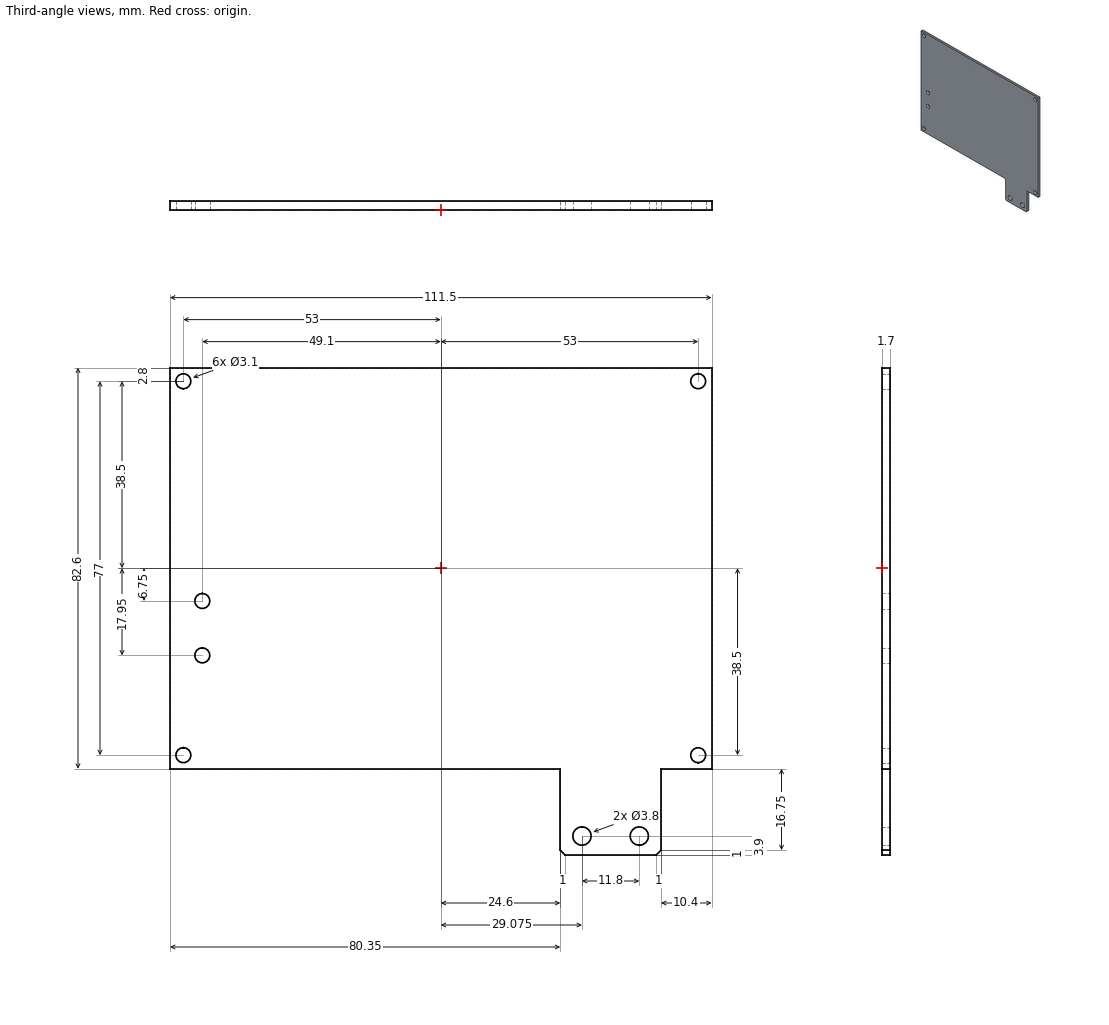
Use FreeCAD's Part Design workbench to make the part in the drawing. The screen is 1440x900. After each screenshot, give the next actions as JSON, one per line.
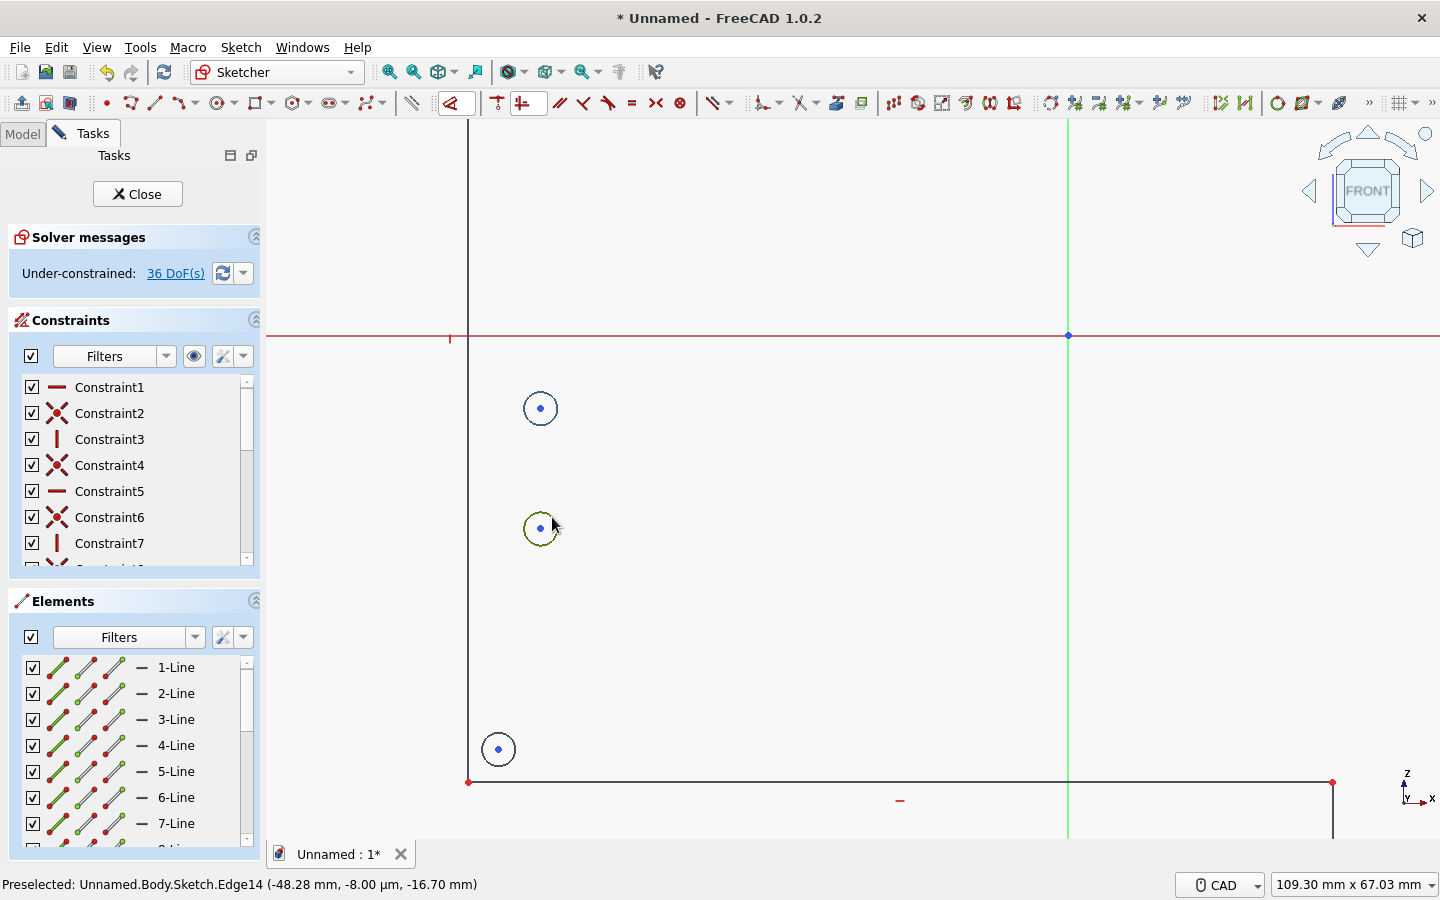
{"action": "left_click", "coordinate": [510, 738]}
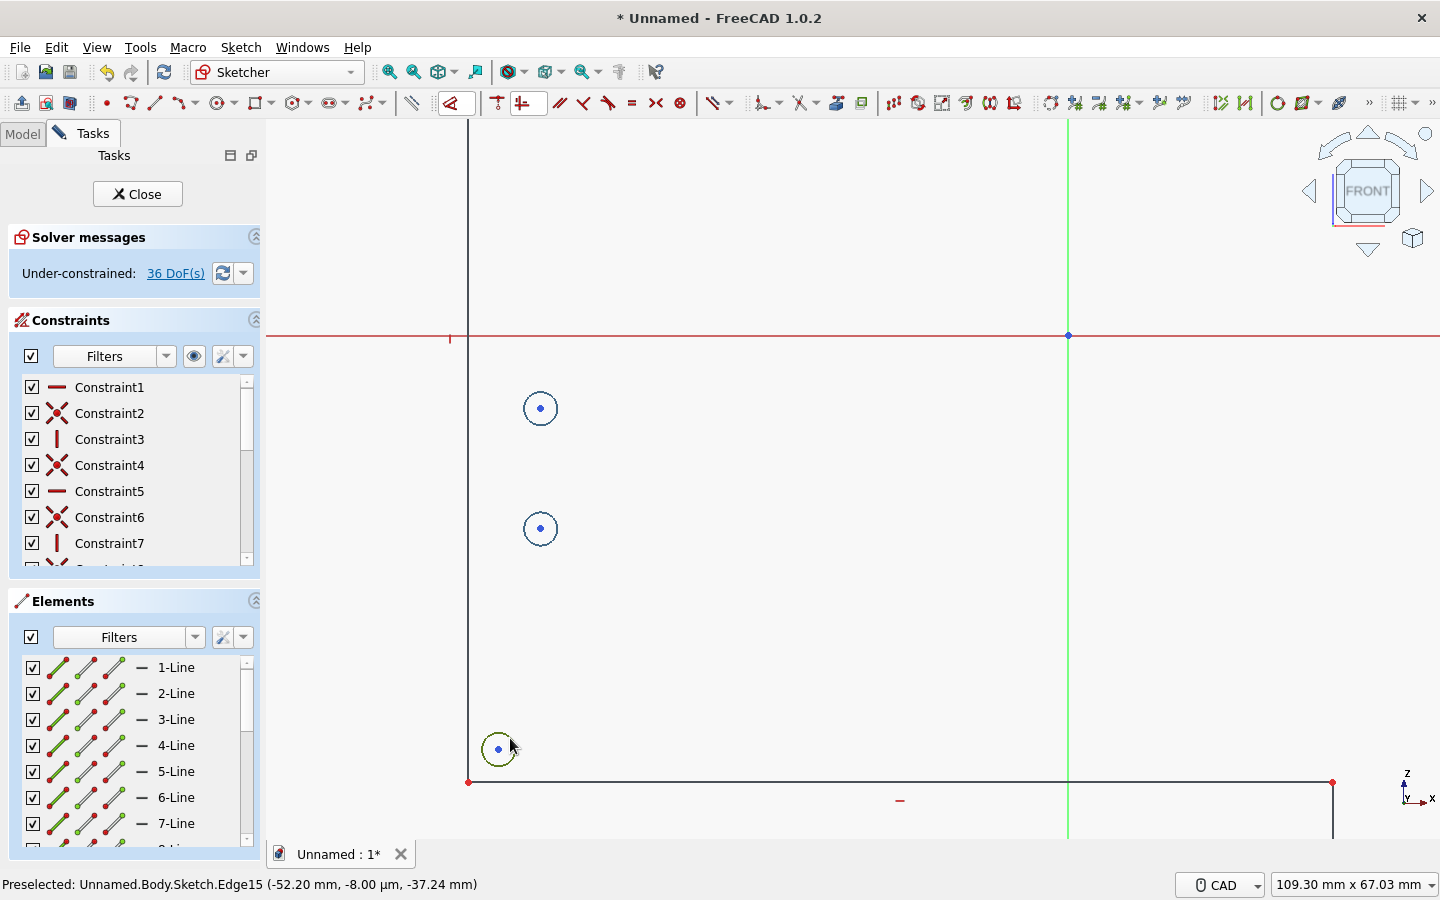
{"action": "scroll", "coordinate": [553, 518], "scroll_direction": "down", "scroll_amount": 4}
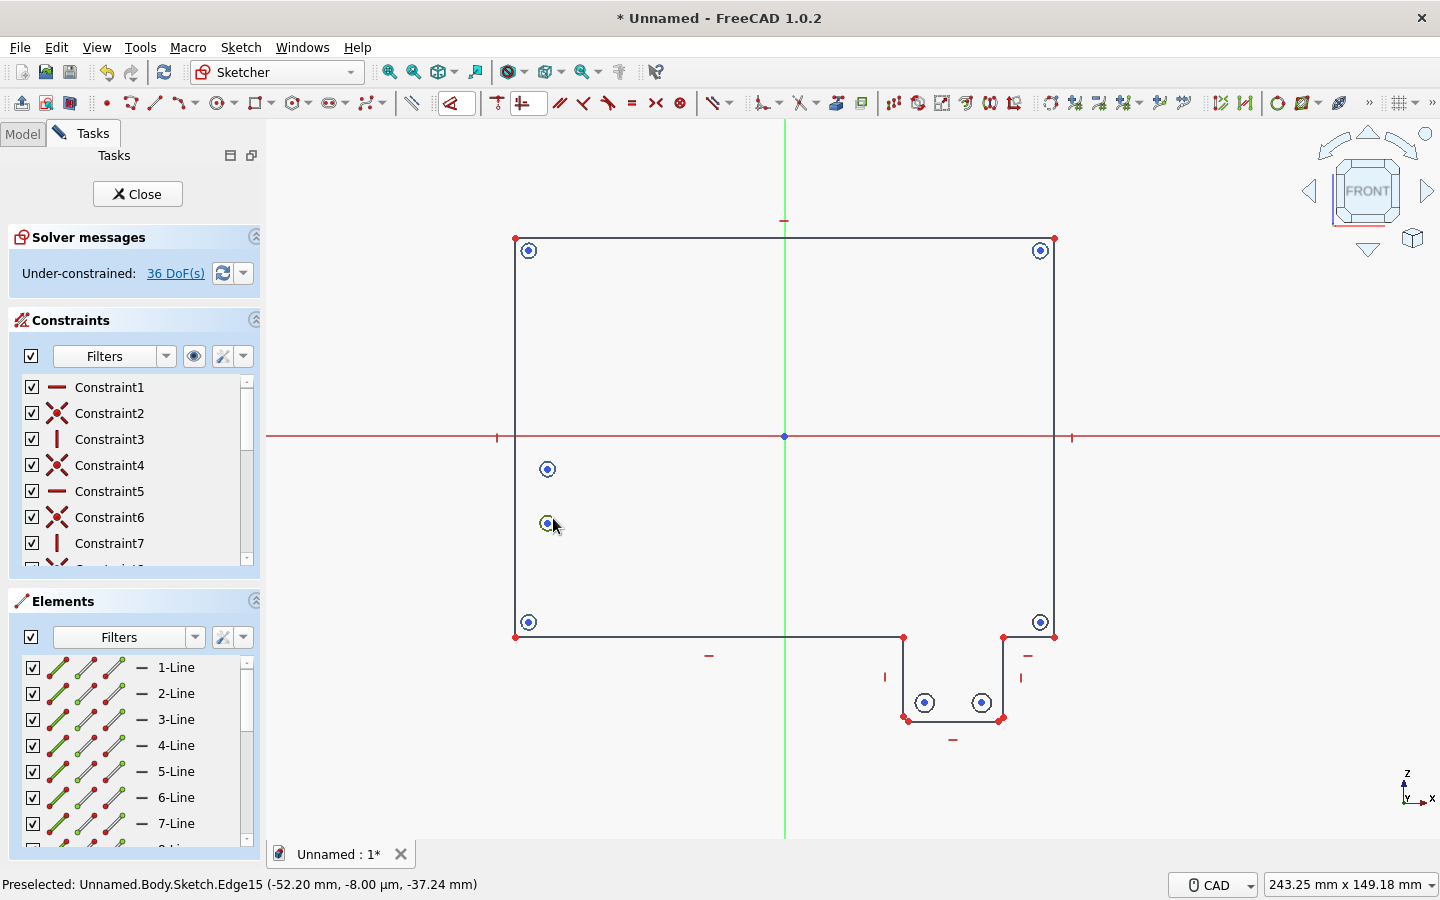
{"action": "scroll", "coordinate": [1046, 617], "scroll_direction": "up", "scroll_amount": 4}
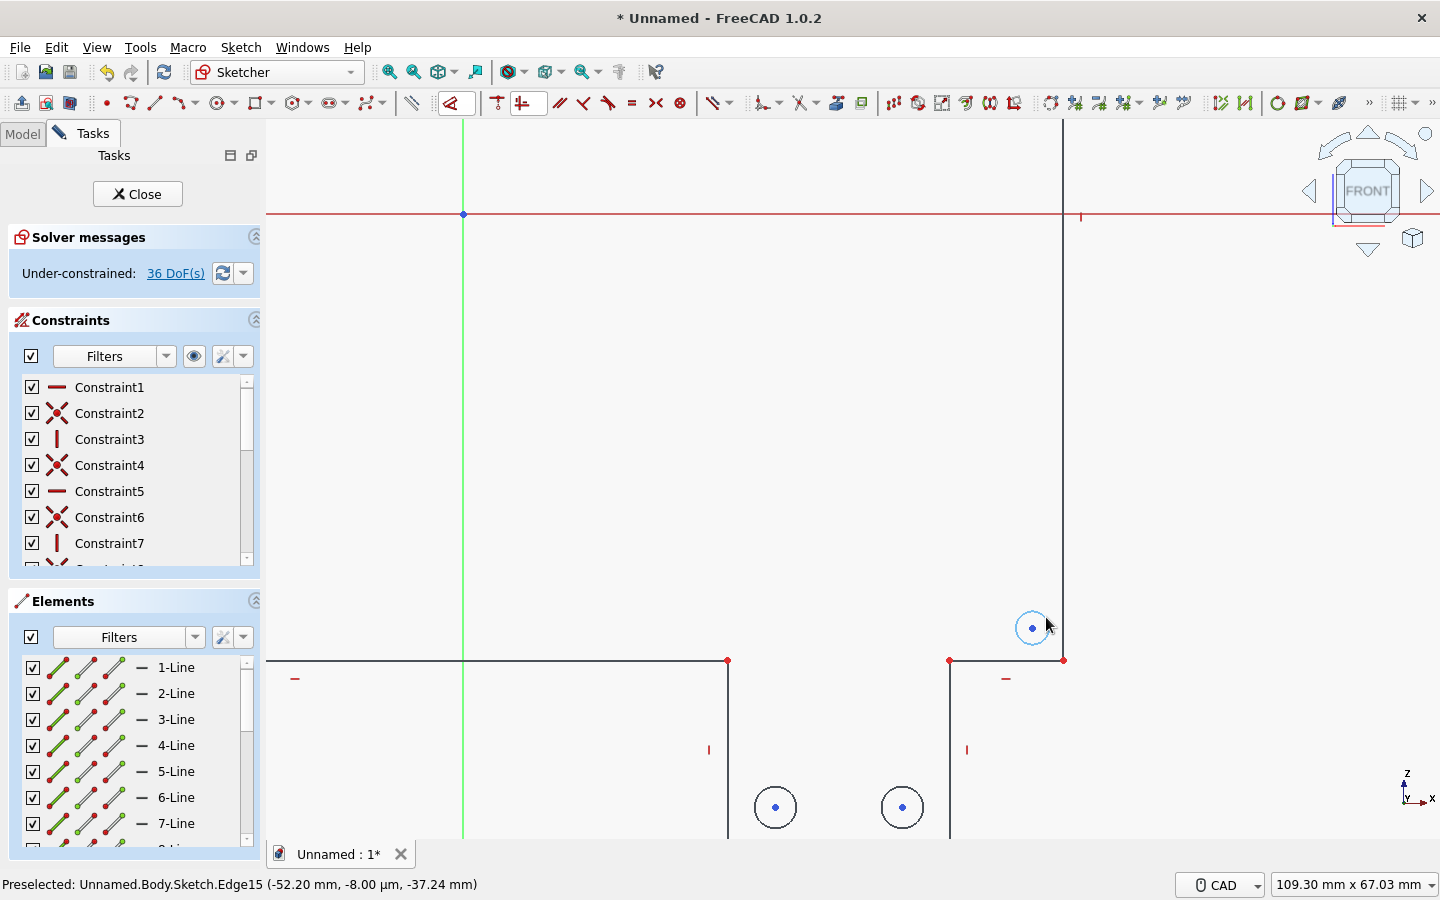
{"action": "left_click", "coordinate": [1044, 616]}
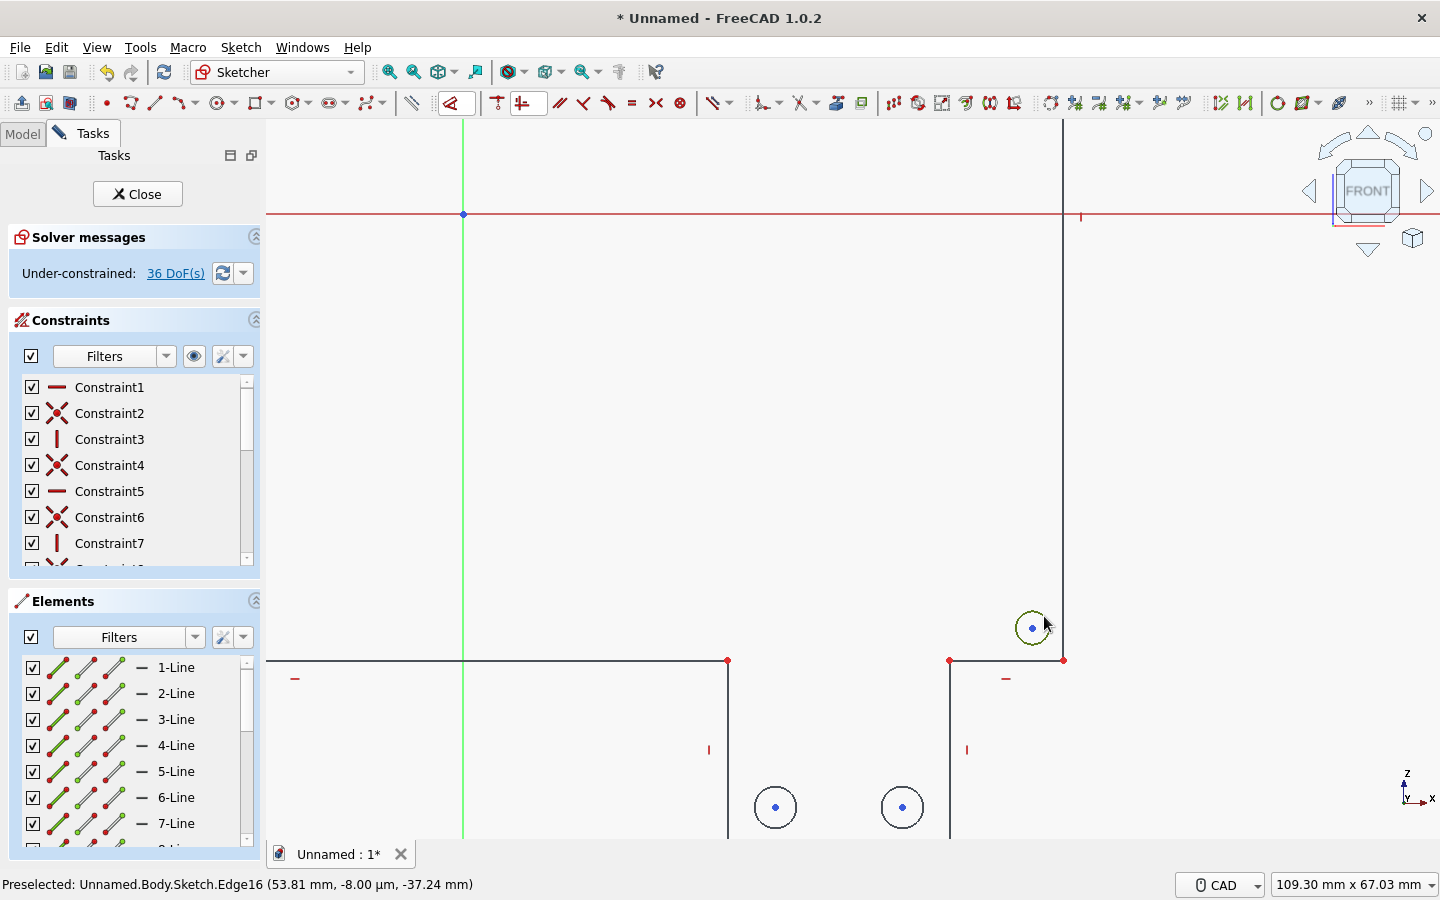
{"action": "key", "text": "e"}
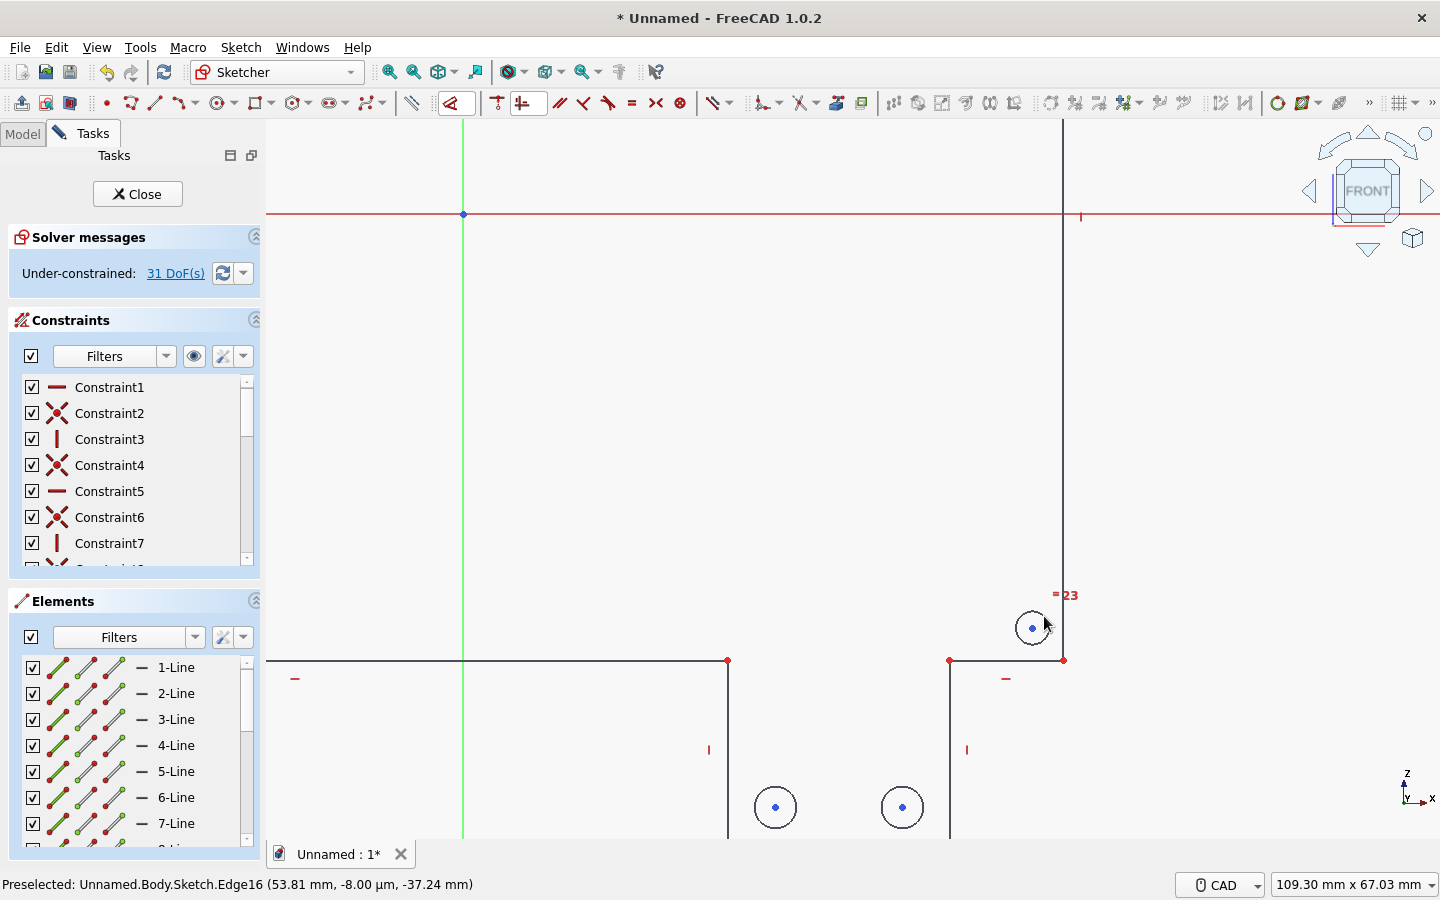
{"action": "left_click", "coordinate": [790, 793]}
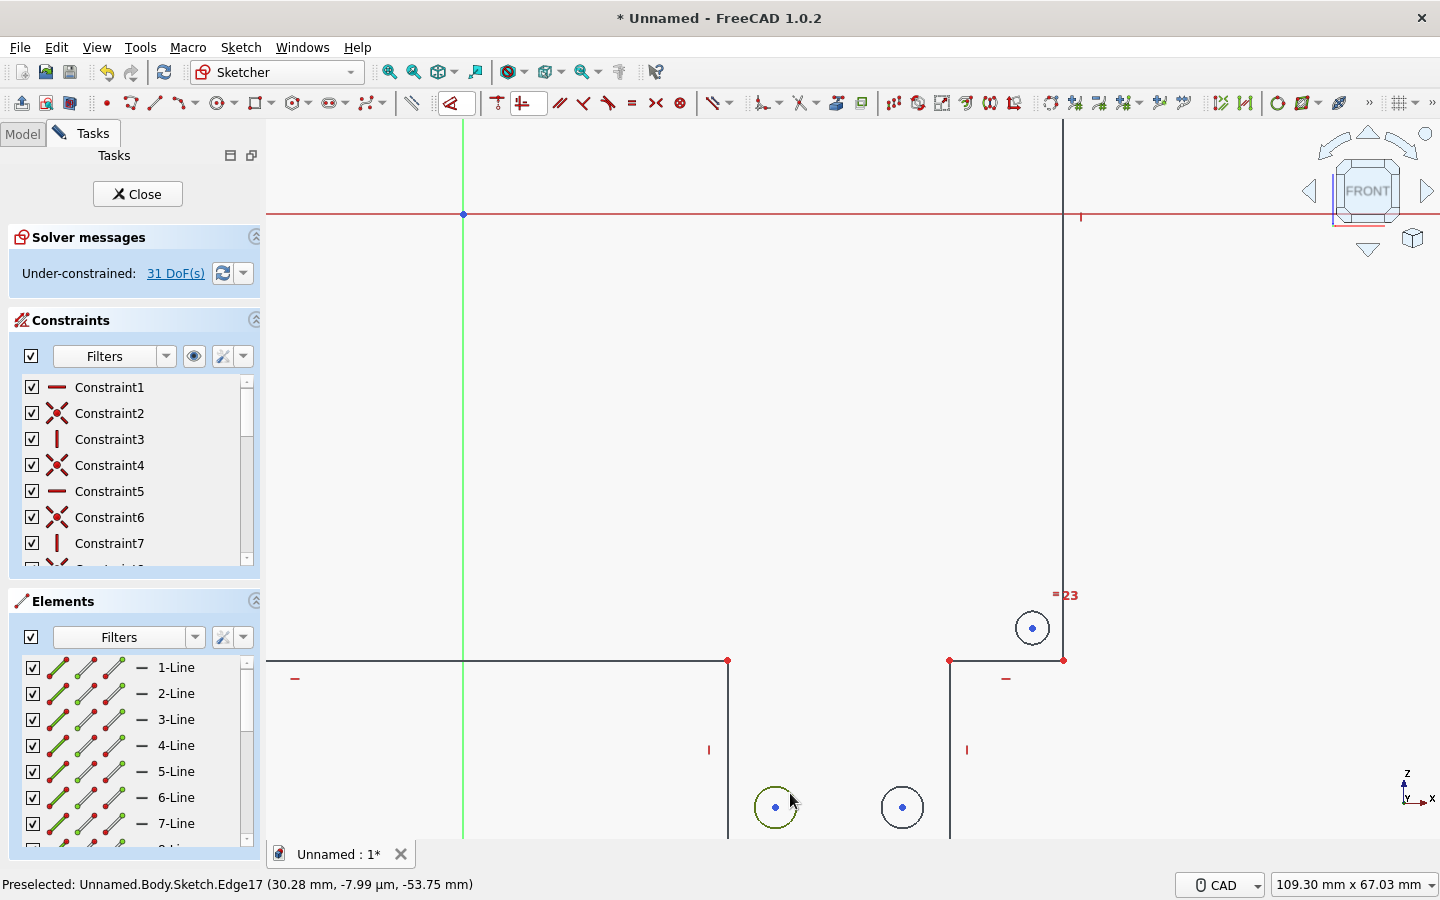
{"action": "left_click", "coordinate": [917, 793]}